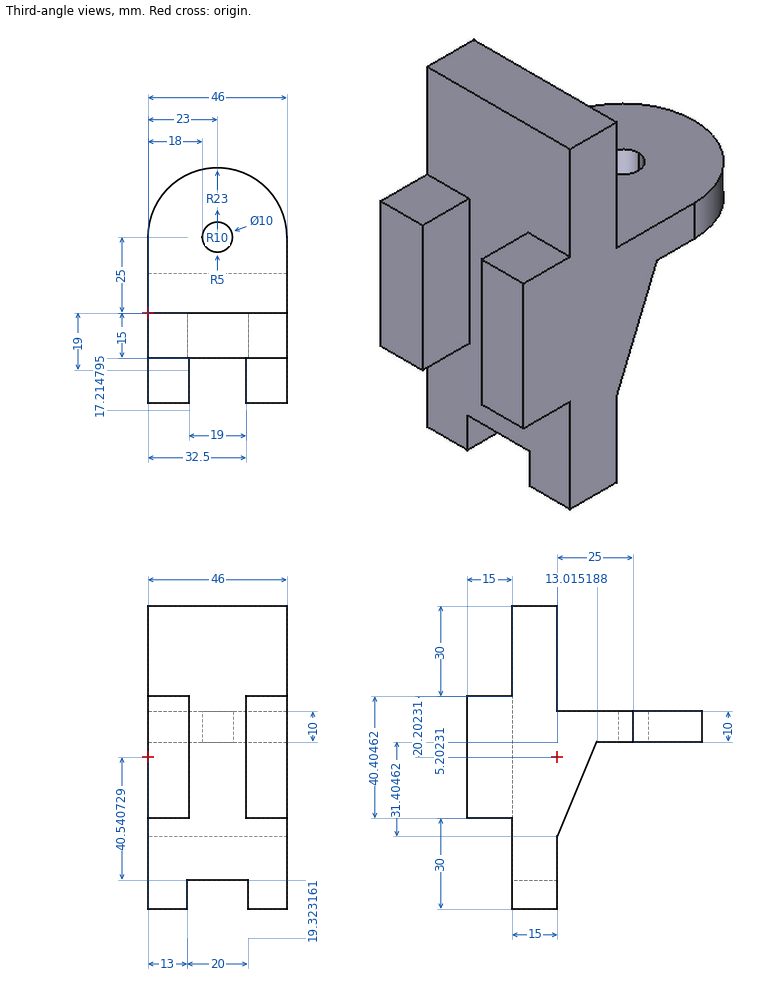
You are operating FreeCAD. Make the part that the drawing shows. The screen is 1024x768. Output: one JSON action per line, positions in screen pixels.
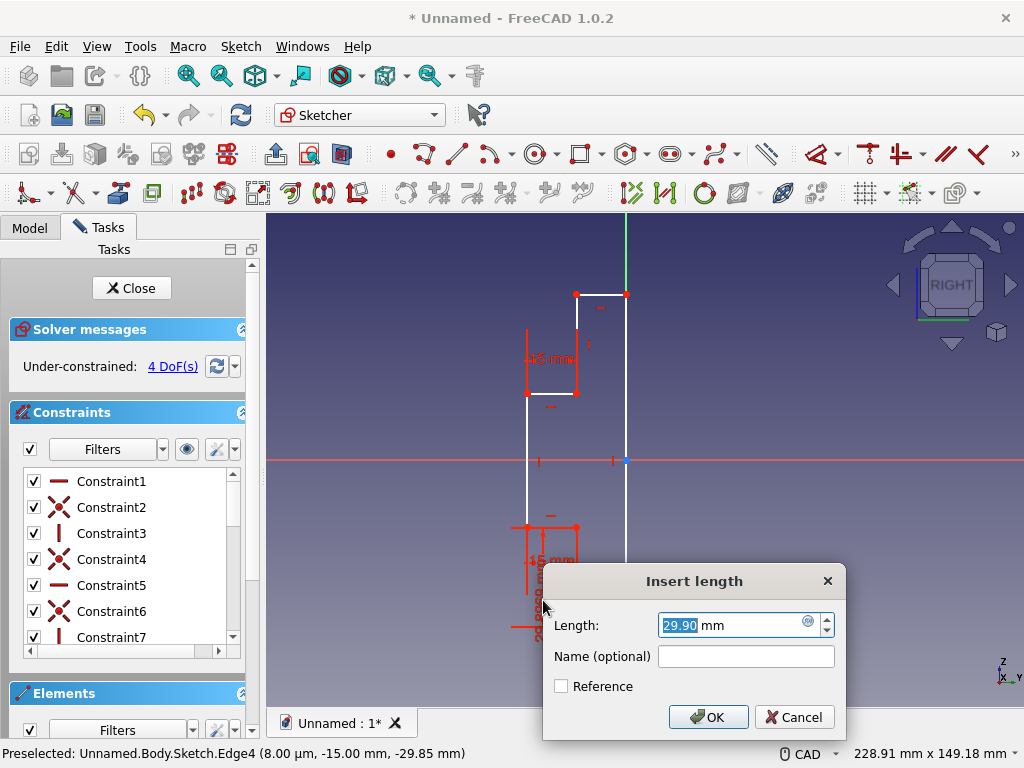
{"action": "type", "text": "30"}
{"action": "key", "text": "Return"}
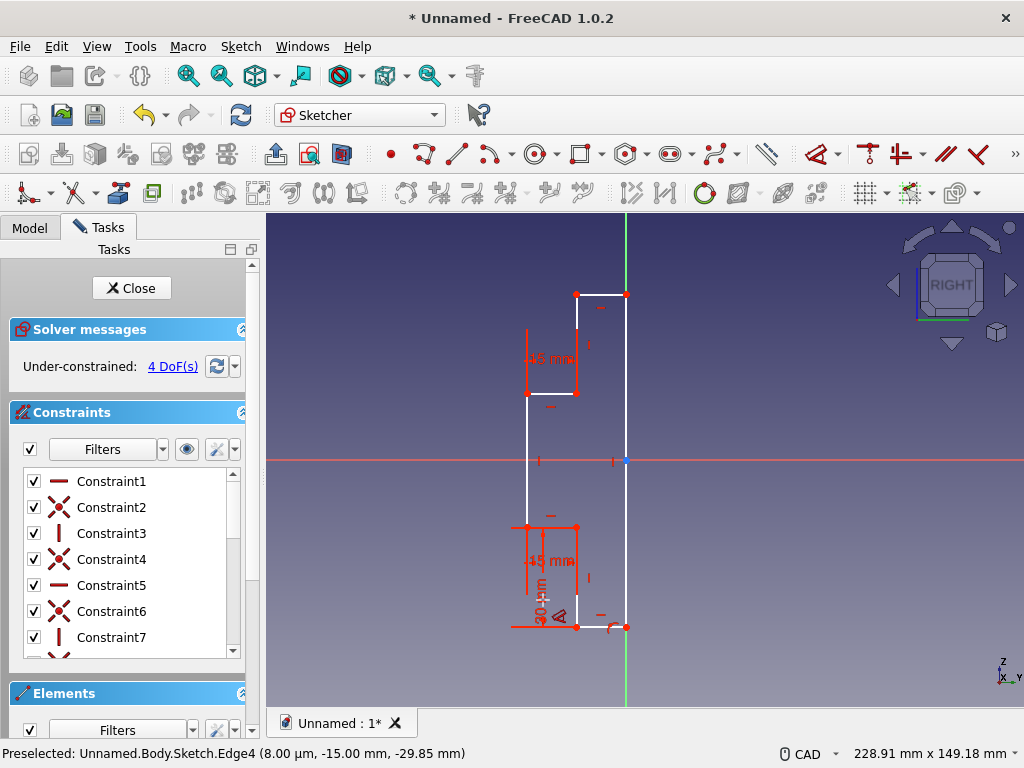
{"action": "left_click", "coordinate": [592, 627]}
{"action": "left_click", "coordinate": [602, 661]}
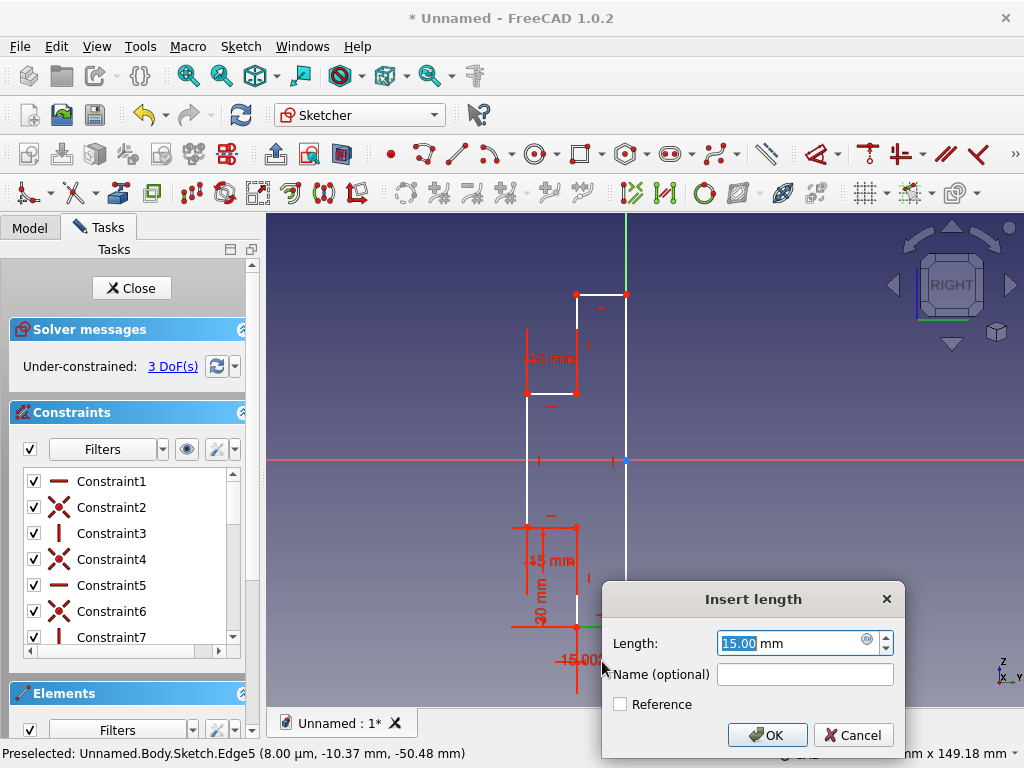
{"action": "type", "text": "15"}
{"action": "key", "text": "Return"}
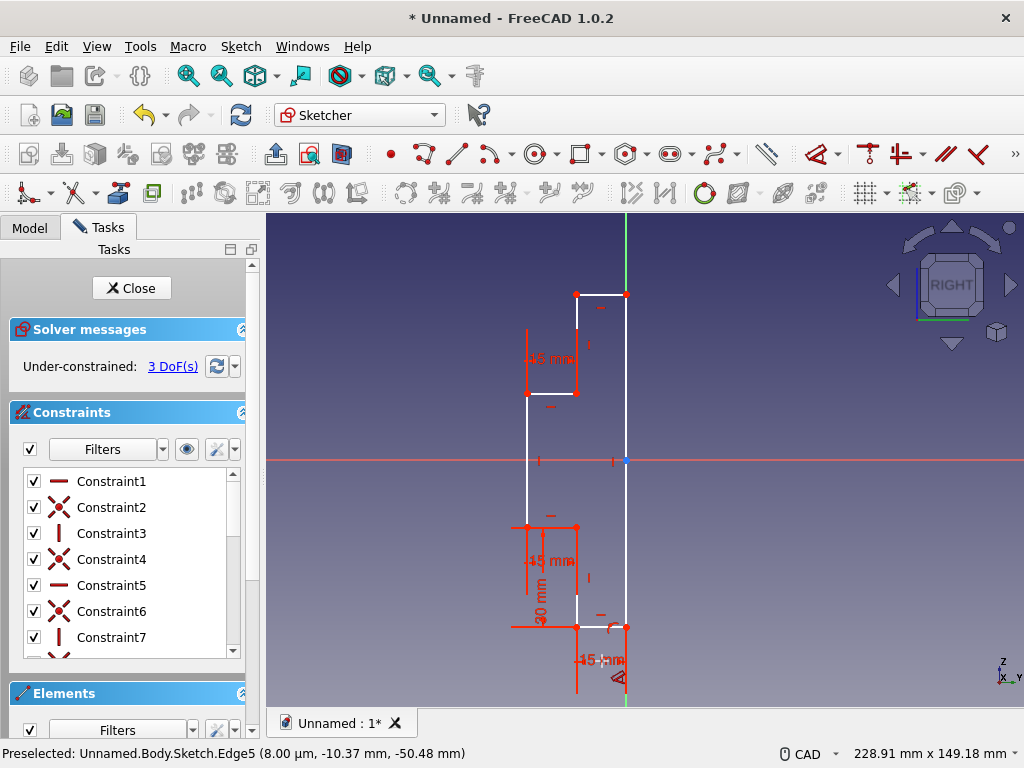
{"action": "left_click", "coordinate": [577, 325]}
{"action": "left_click", "coordinate": [611, 322]}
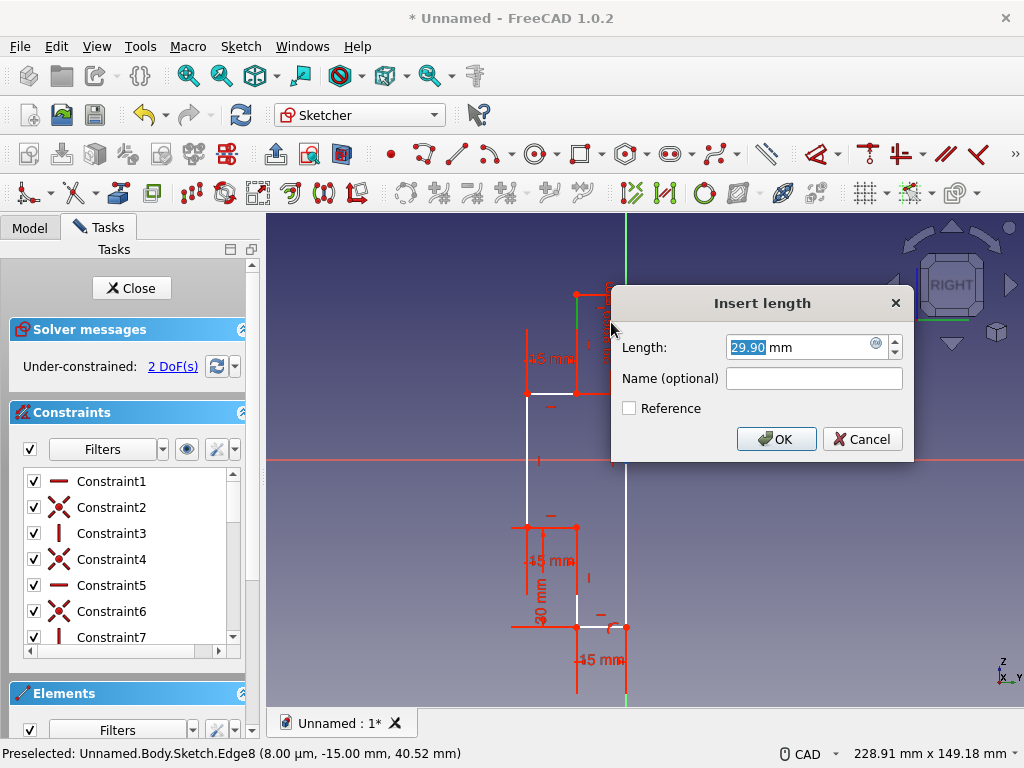
{"action": "type", "text": "30"}
{"action": "key", "text": "Return"}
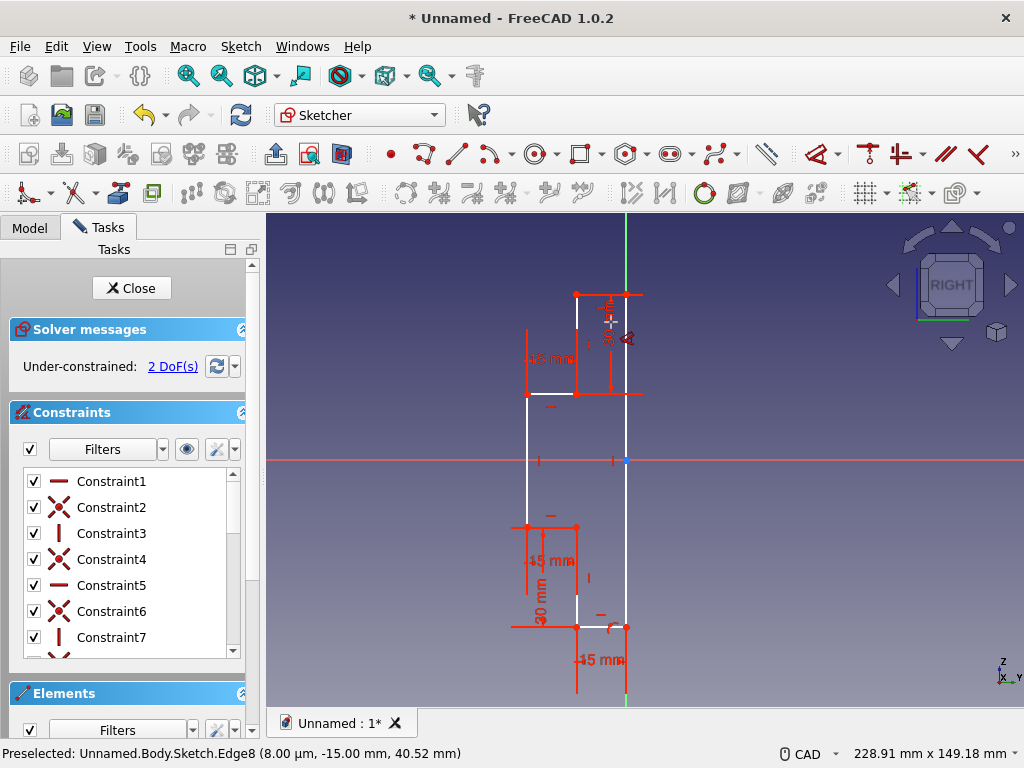
{"action": "left_click", "coordinate": [527, 434]}
{"action": "left_click", "coordinate": [493, 430]}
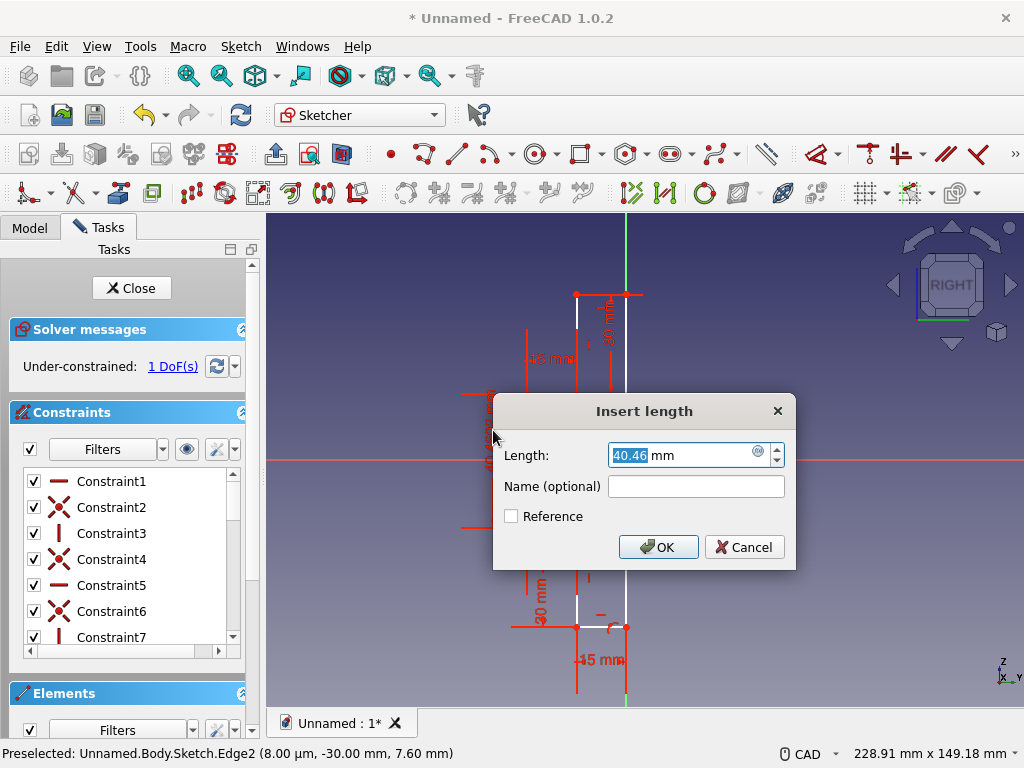
{"action": "type", "text": "40.40462"}
{"action": "key", "text": "Return"}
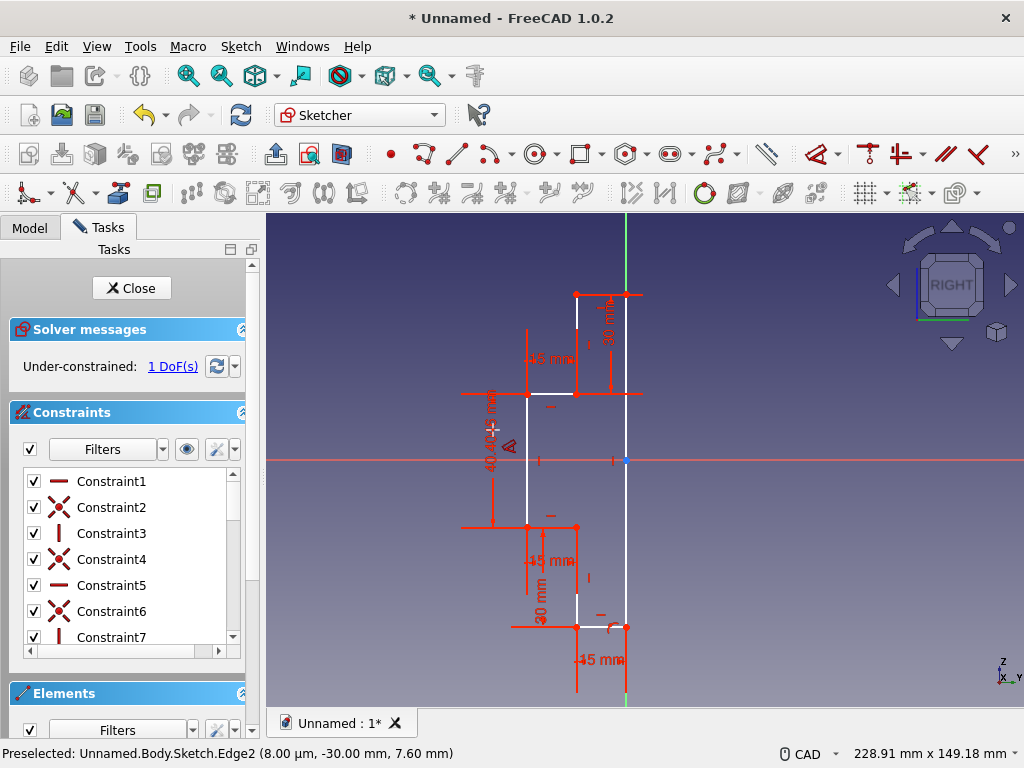
{"action": "left_click", "coordinate": [577, 394]}
{"action": "left_click", "coordinate": [660, 427]}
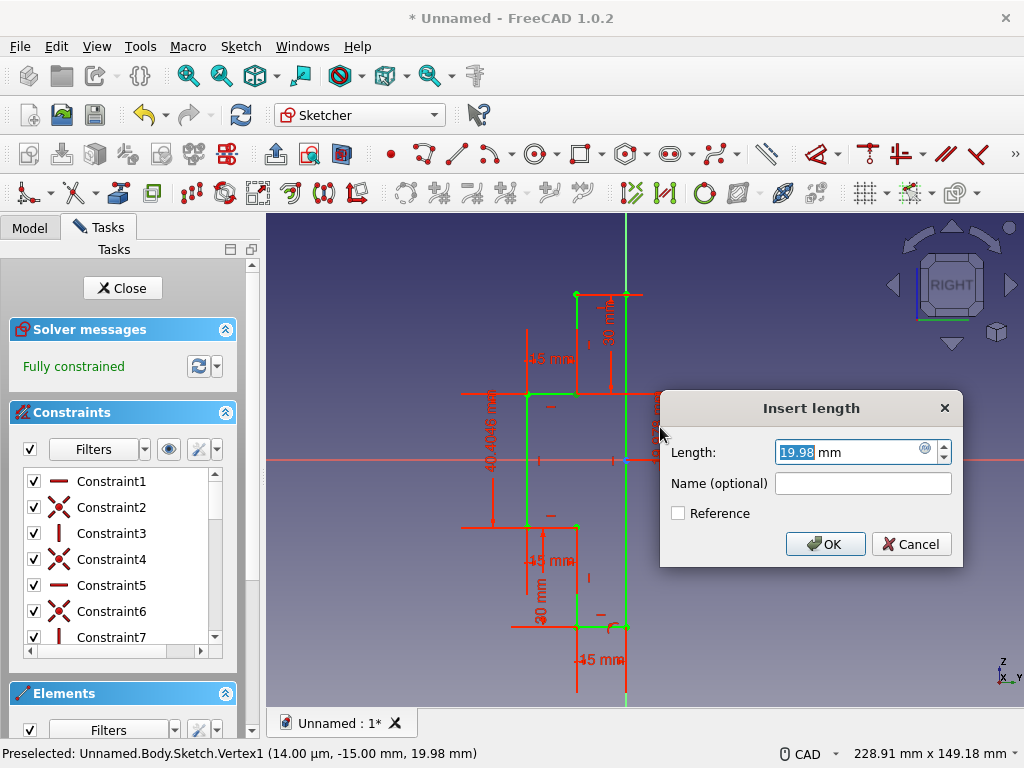
{"action": "type", "text": "20.20231"}
{"action": "key", "text": "Return"}
{"action": "key", "text": "Escape"}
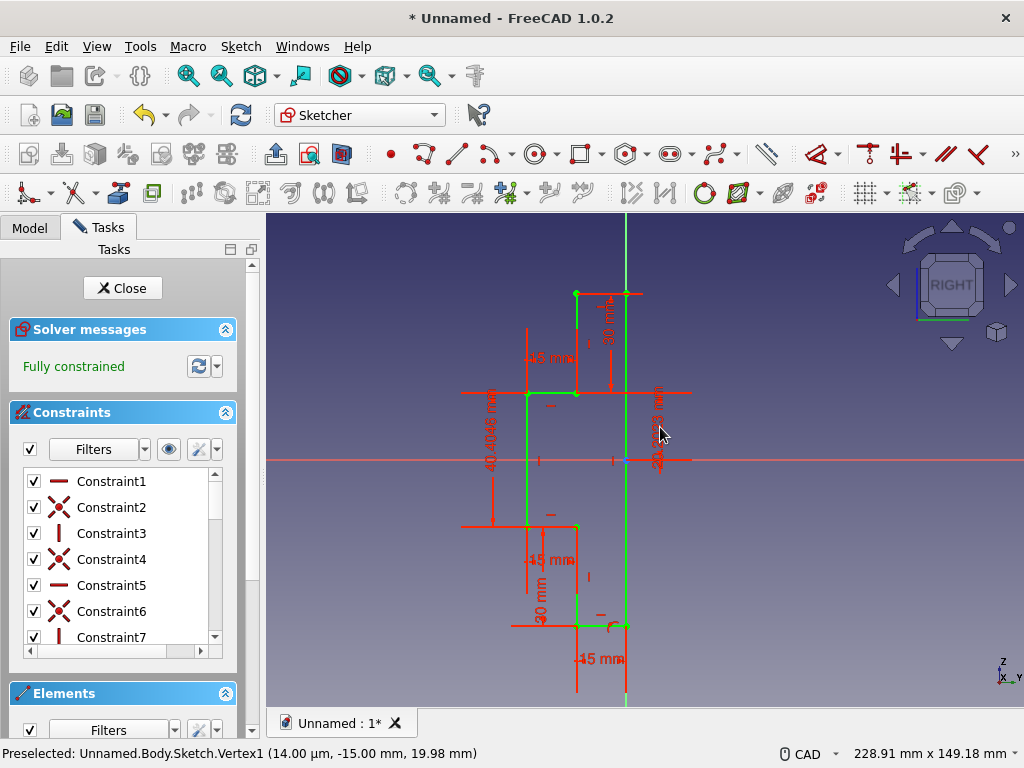
{"action": "left_click", "coordinate": [123, 288]}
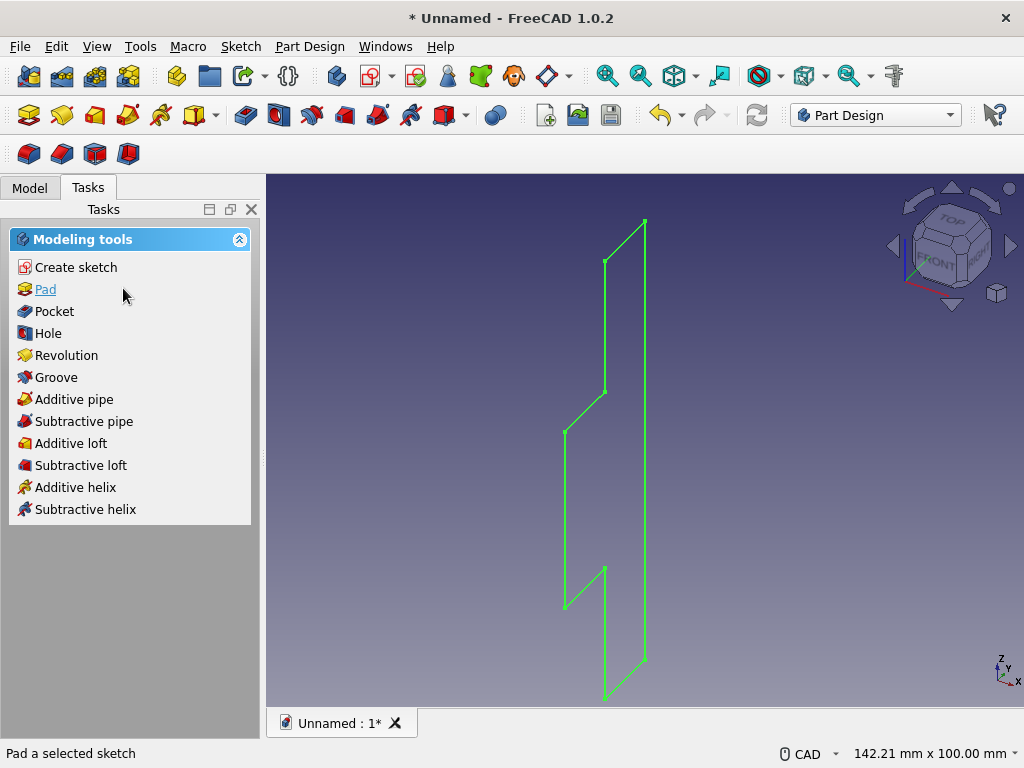
{"action": "left_click", "coordinate": [29, 116]}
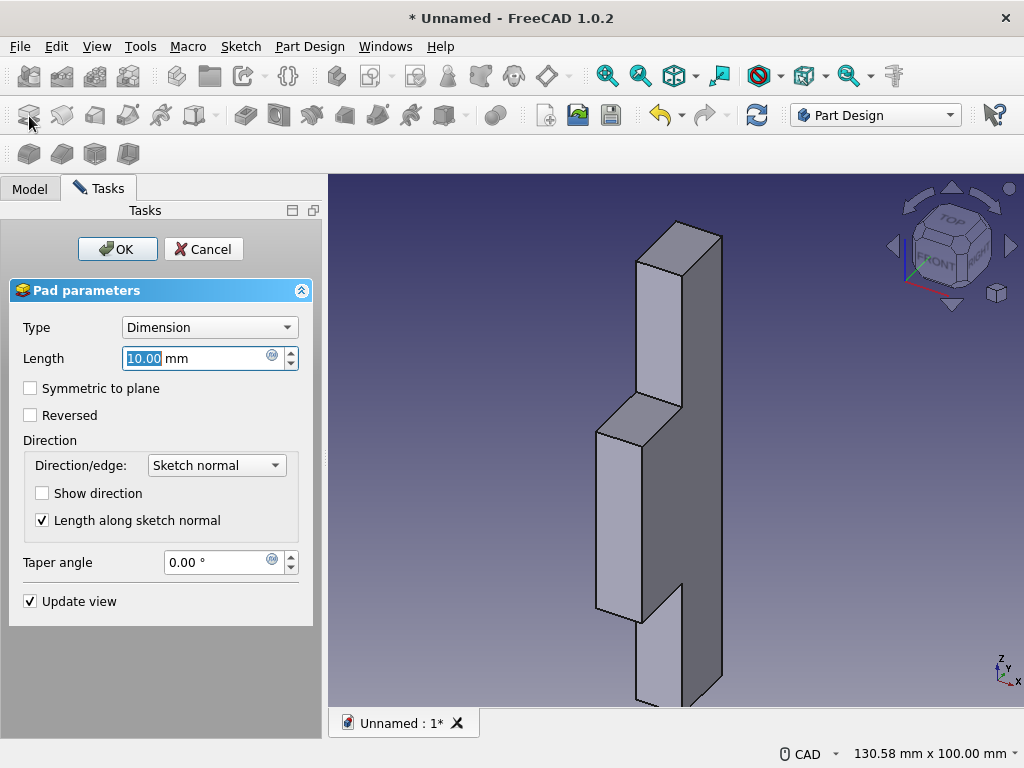
{"action": "type", "text": "46"}
{"action": "key", "text": "Tab"}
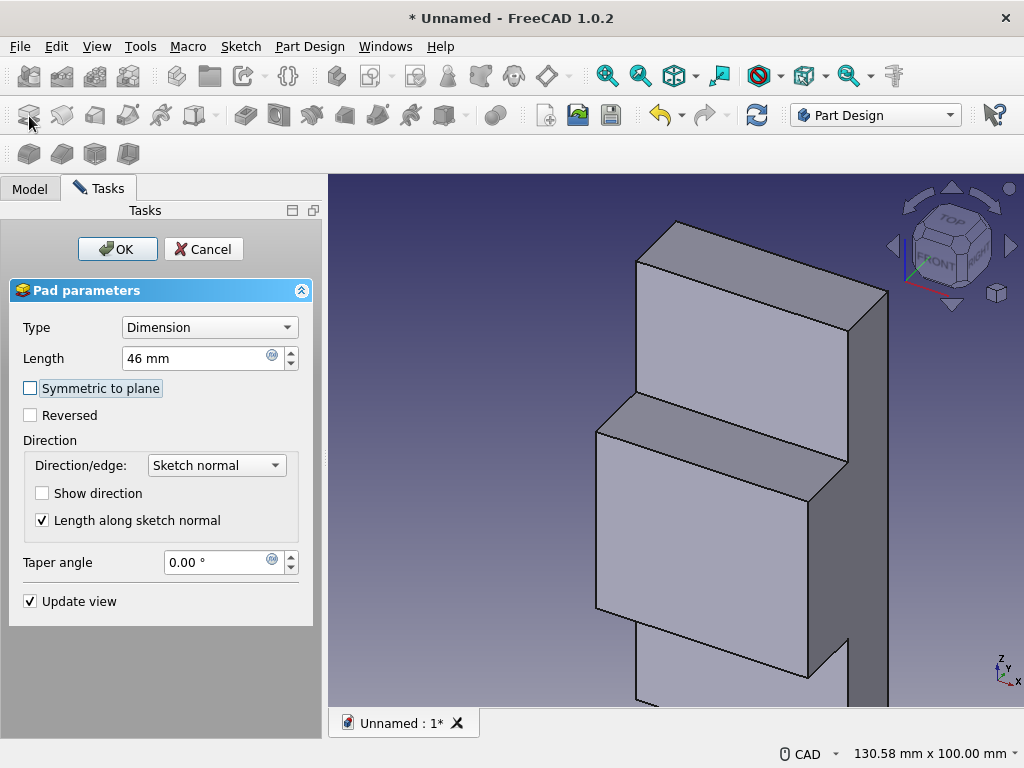
{"action": "left_click", "coordinate": [118, 249]}